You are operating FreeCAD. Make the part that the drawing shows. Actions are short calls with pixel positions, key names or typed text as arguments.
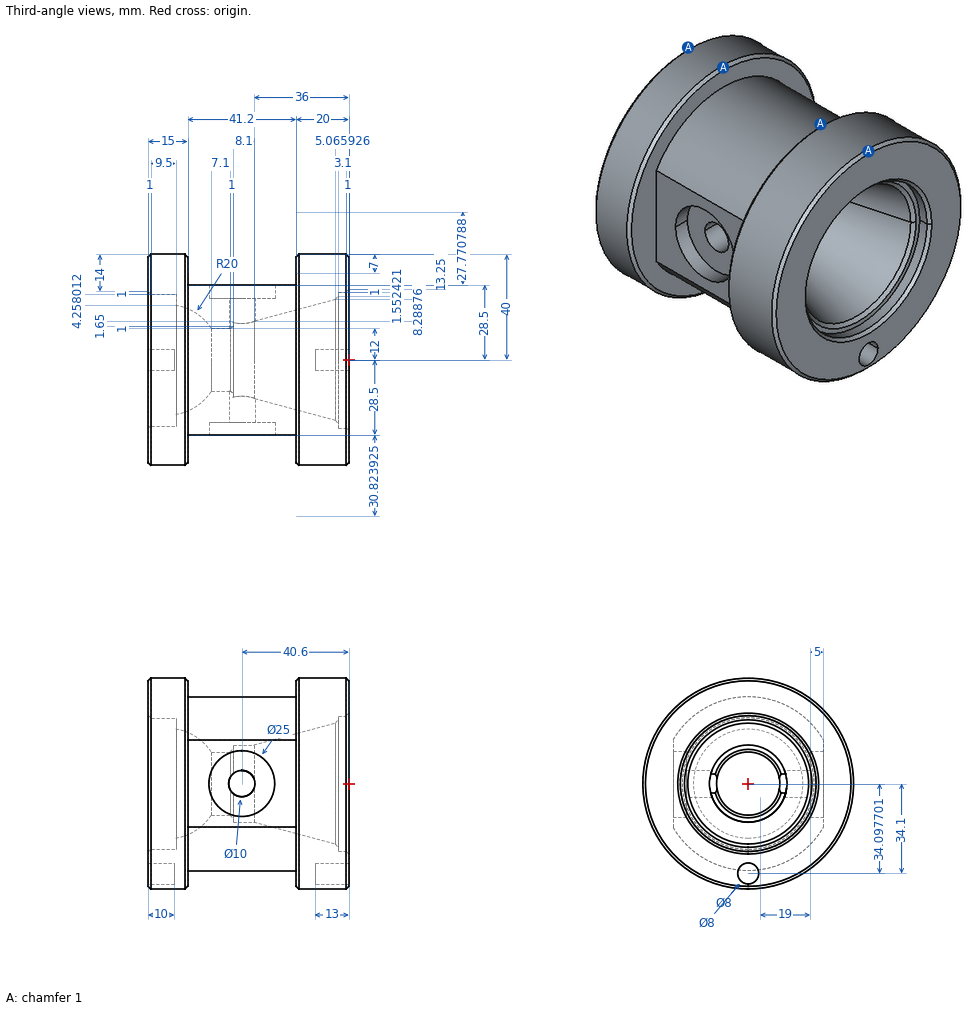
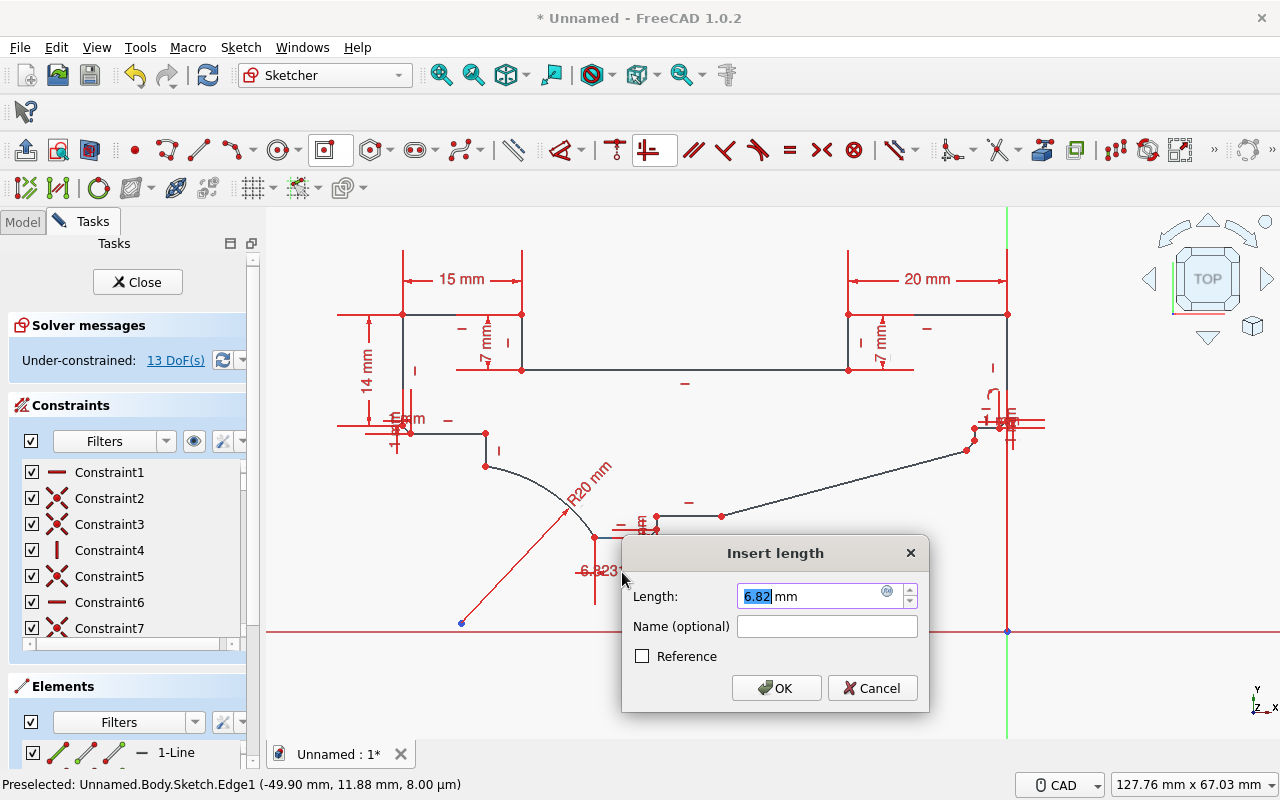
text(7.1)
key(Return)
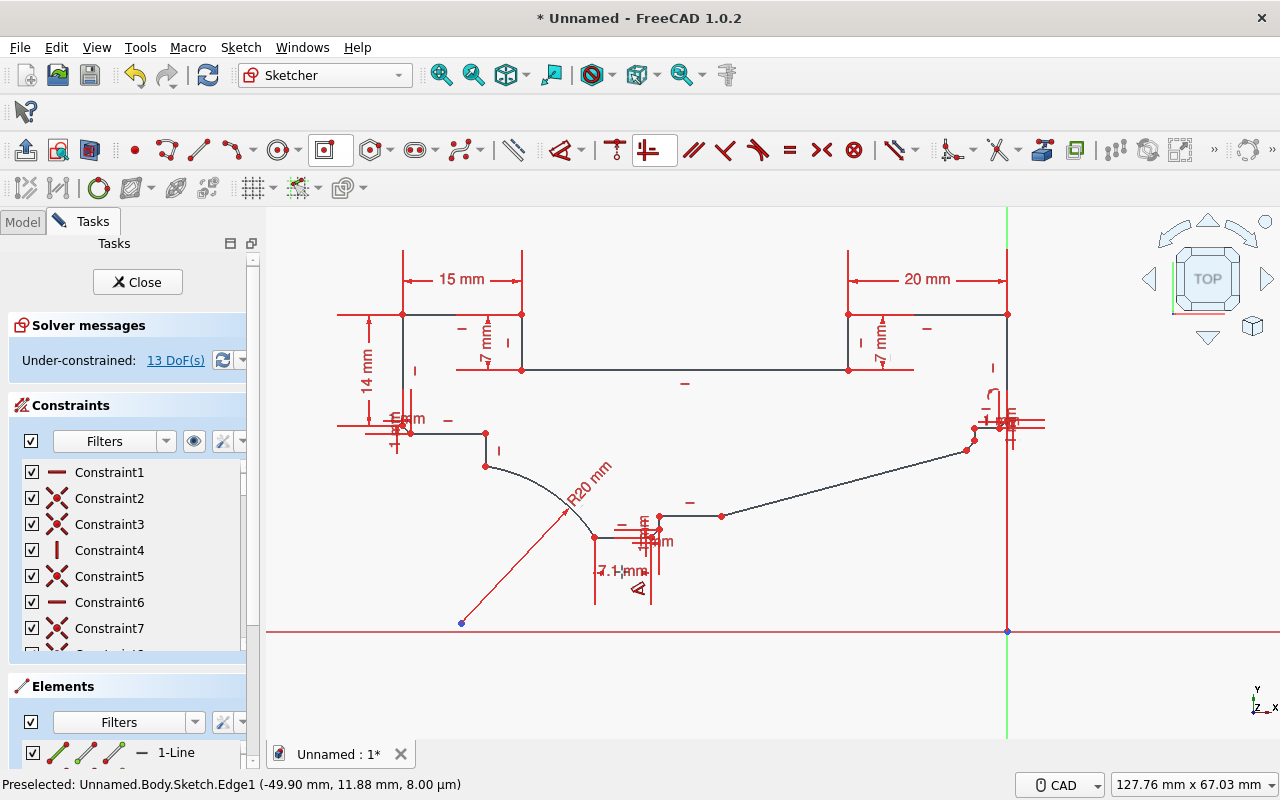
click(678, 516)
click(690, 482)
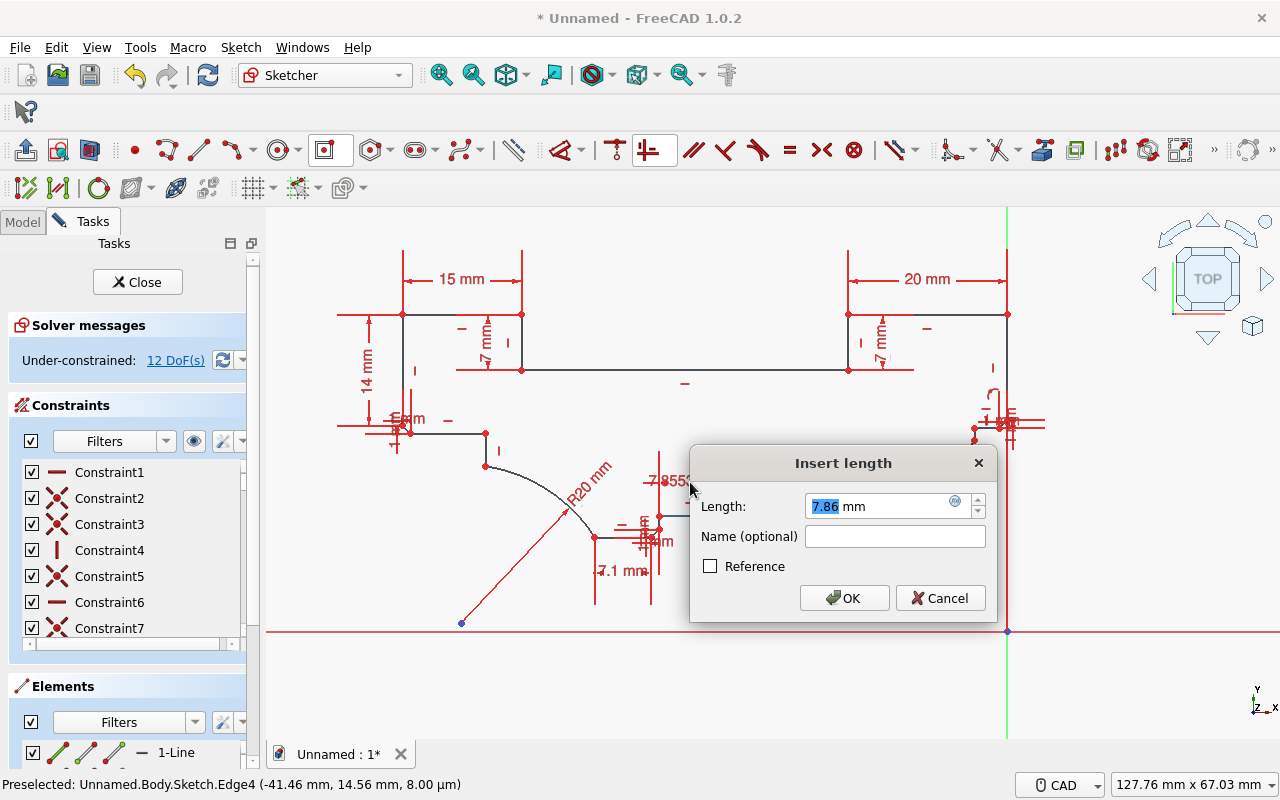
text(8.1)
key(Return)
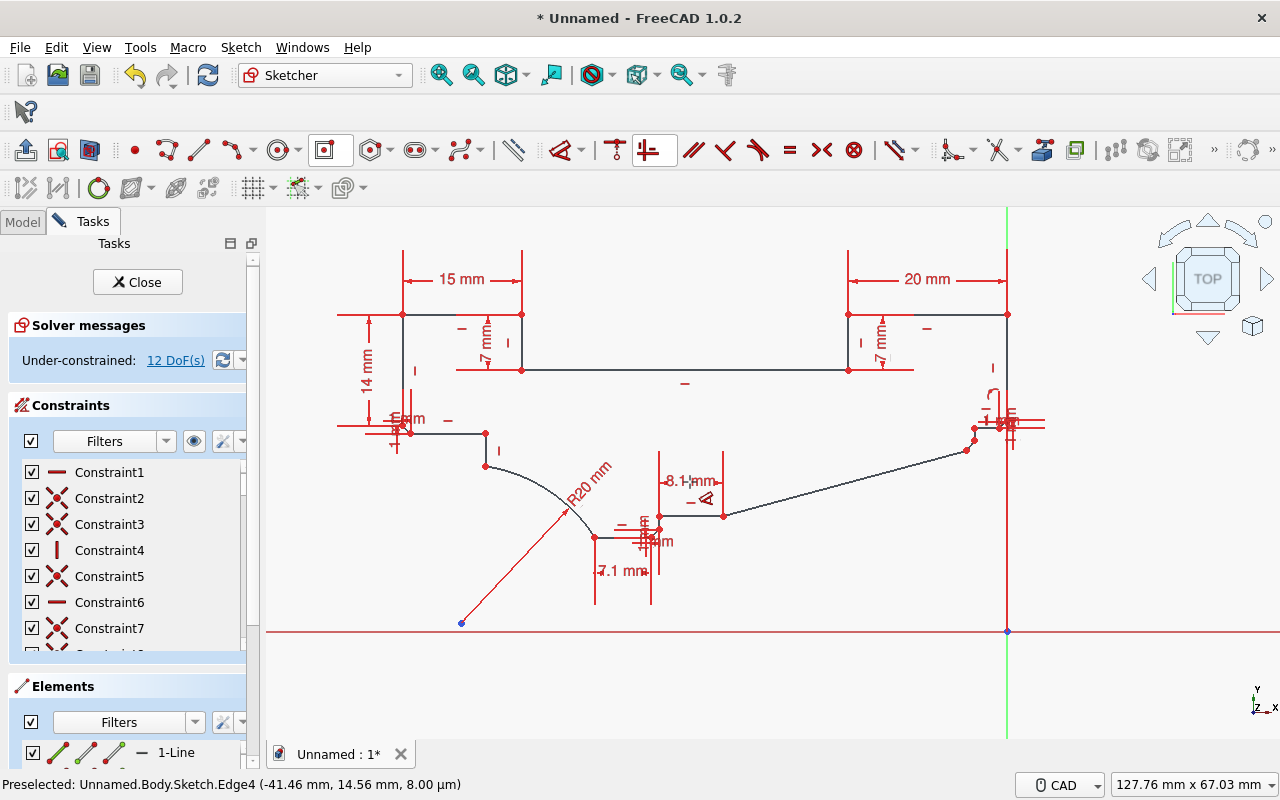
scroll(984, 428, up, 3)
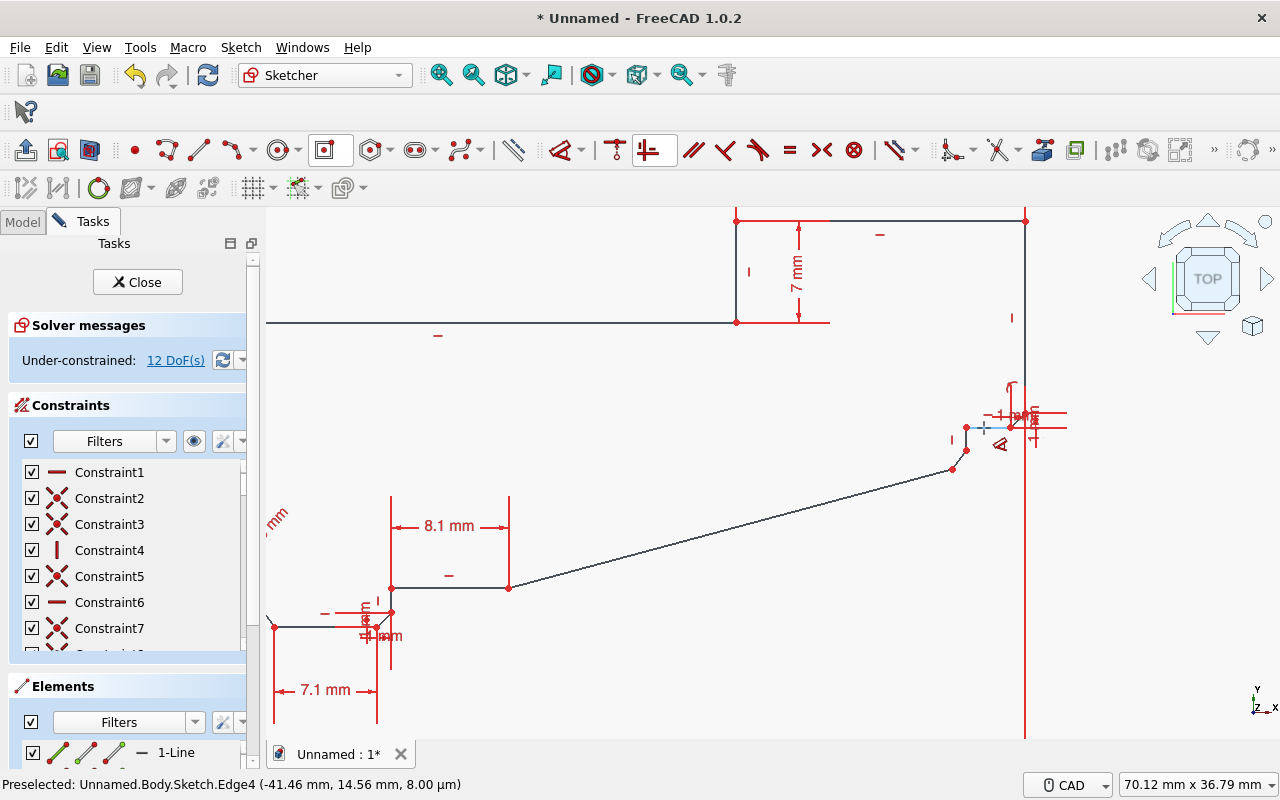
click(984, 428)
click(989, 394)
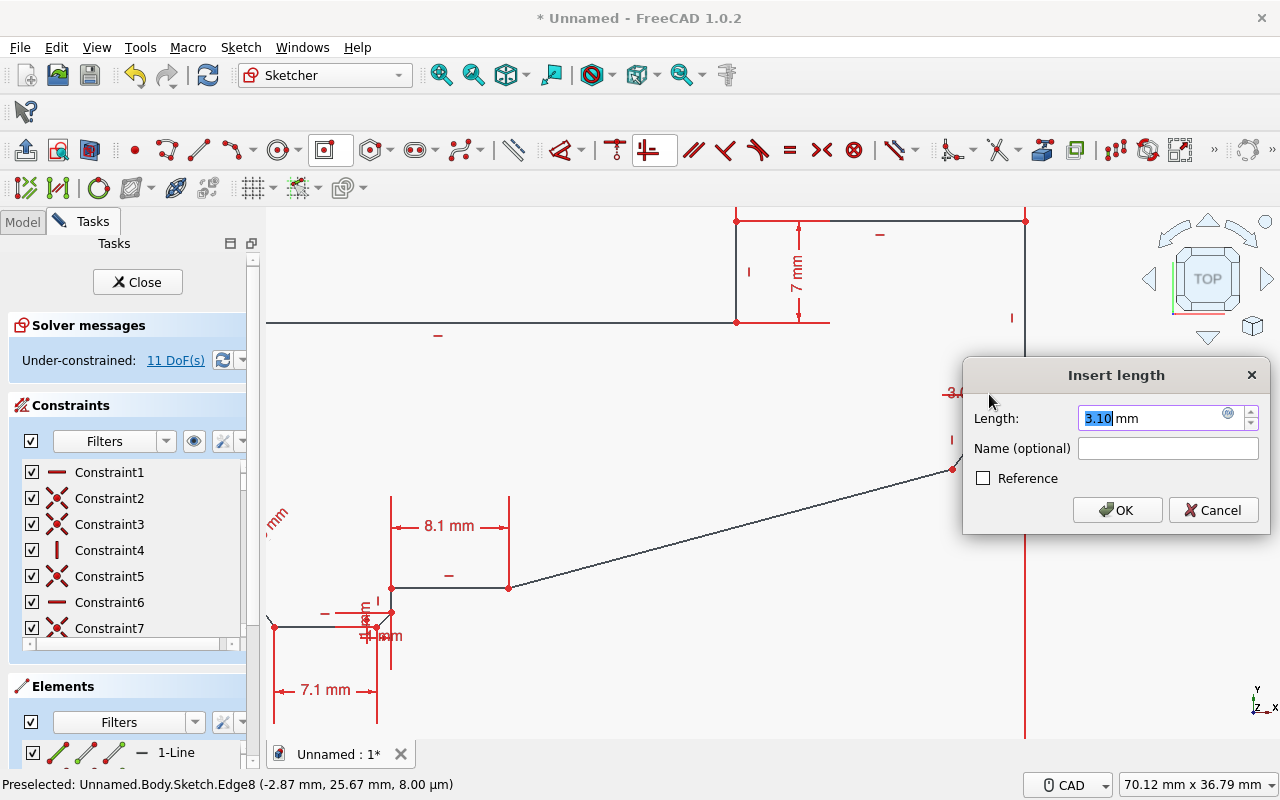
text(3.1)
key(Return)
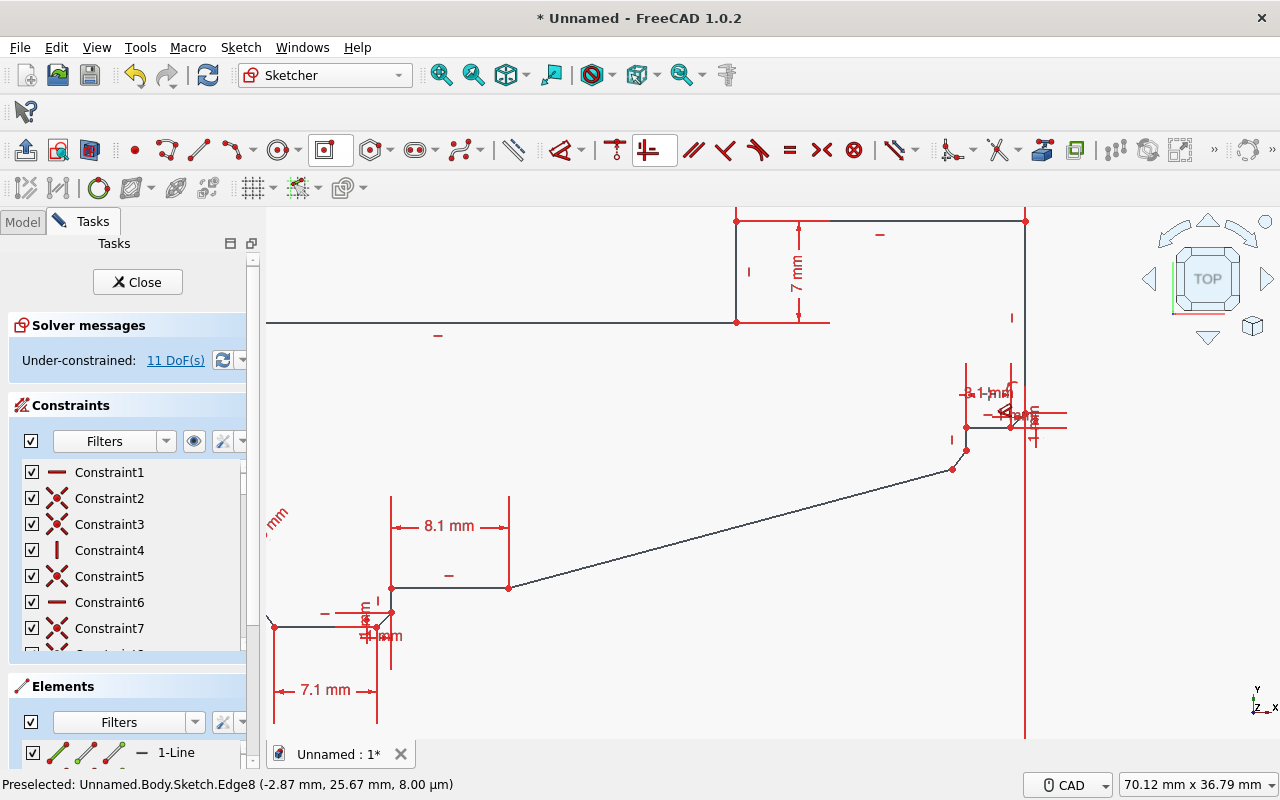
scroll(984, 428, down, 3)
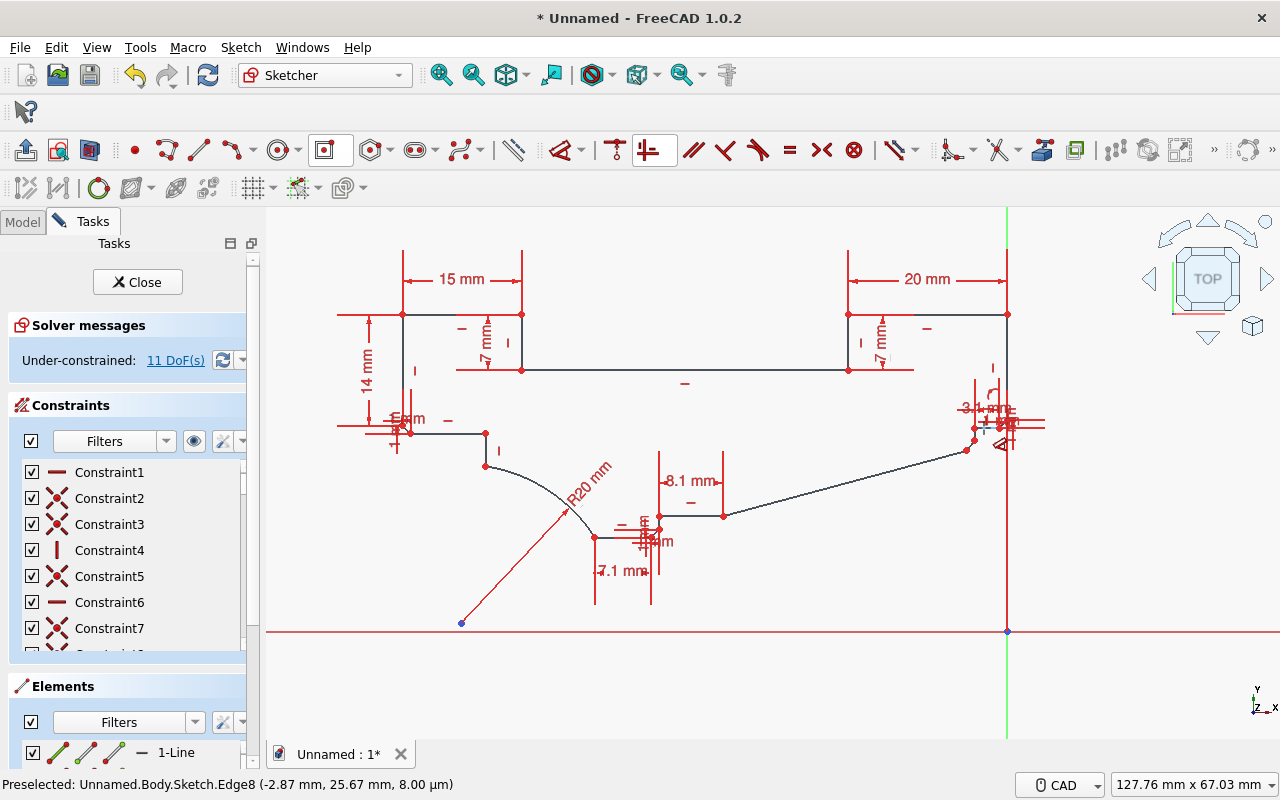
click(433, 434)
click(448, 400)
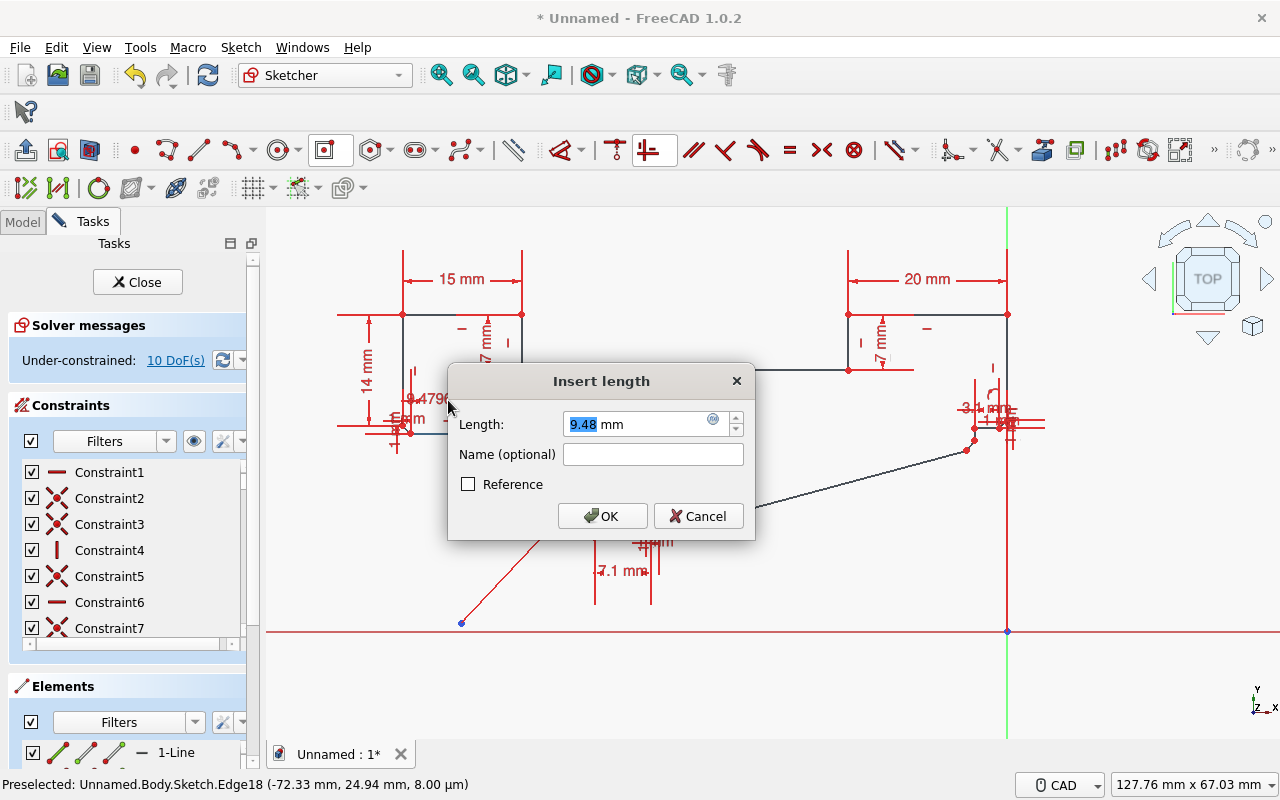
text(9.5)
key(Return)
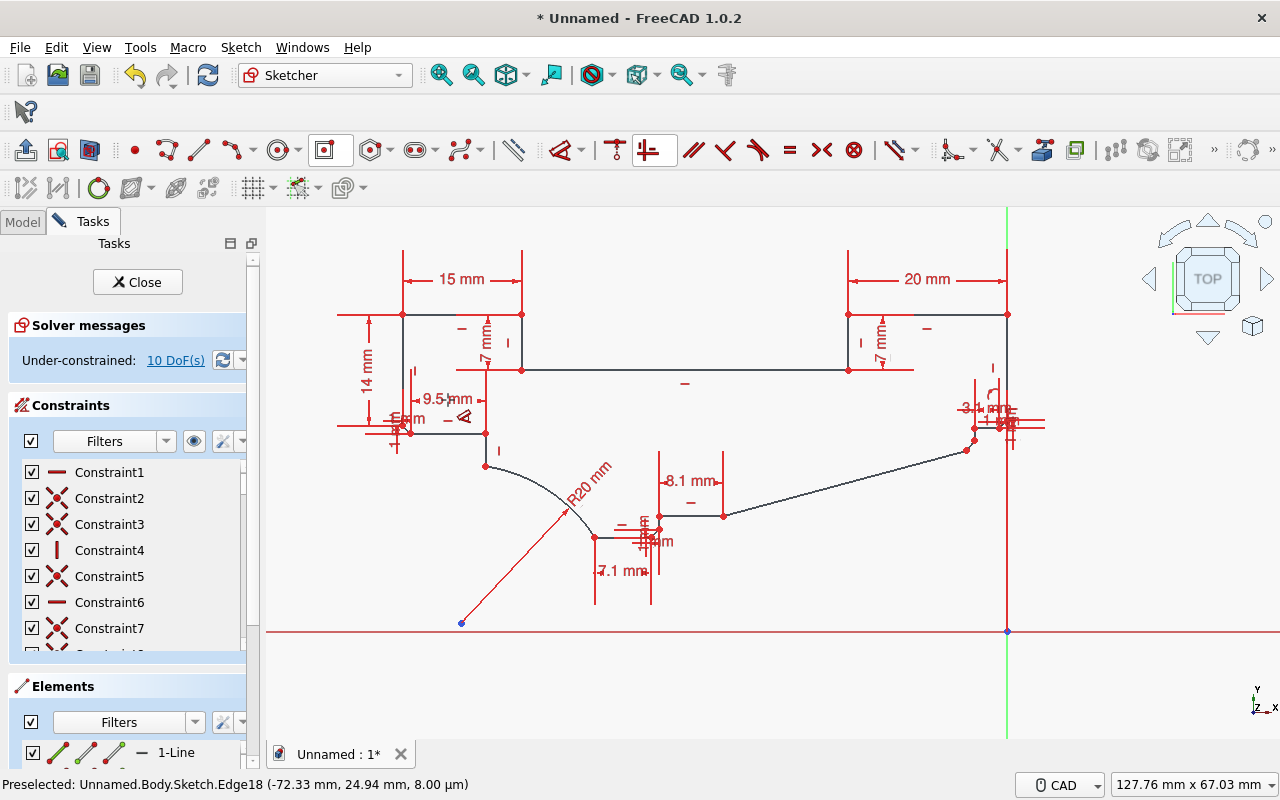
click(595, 538)
click(1041, 585)